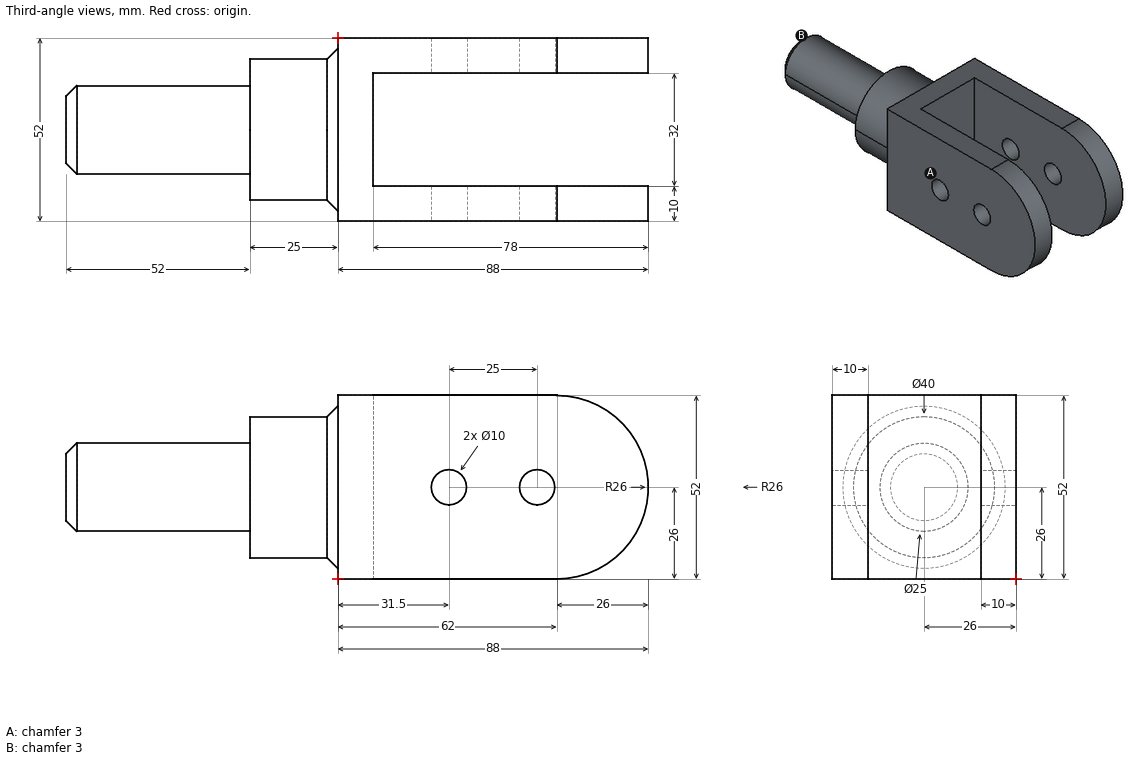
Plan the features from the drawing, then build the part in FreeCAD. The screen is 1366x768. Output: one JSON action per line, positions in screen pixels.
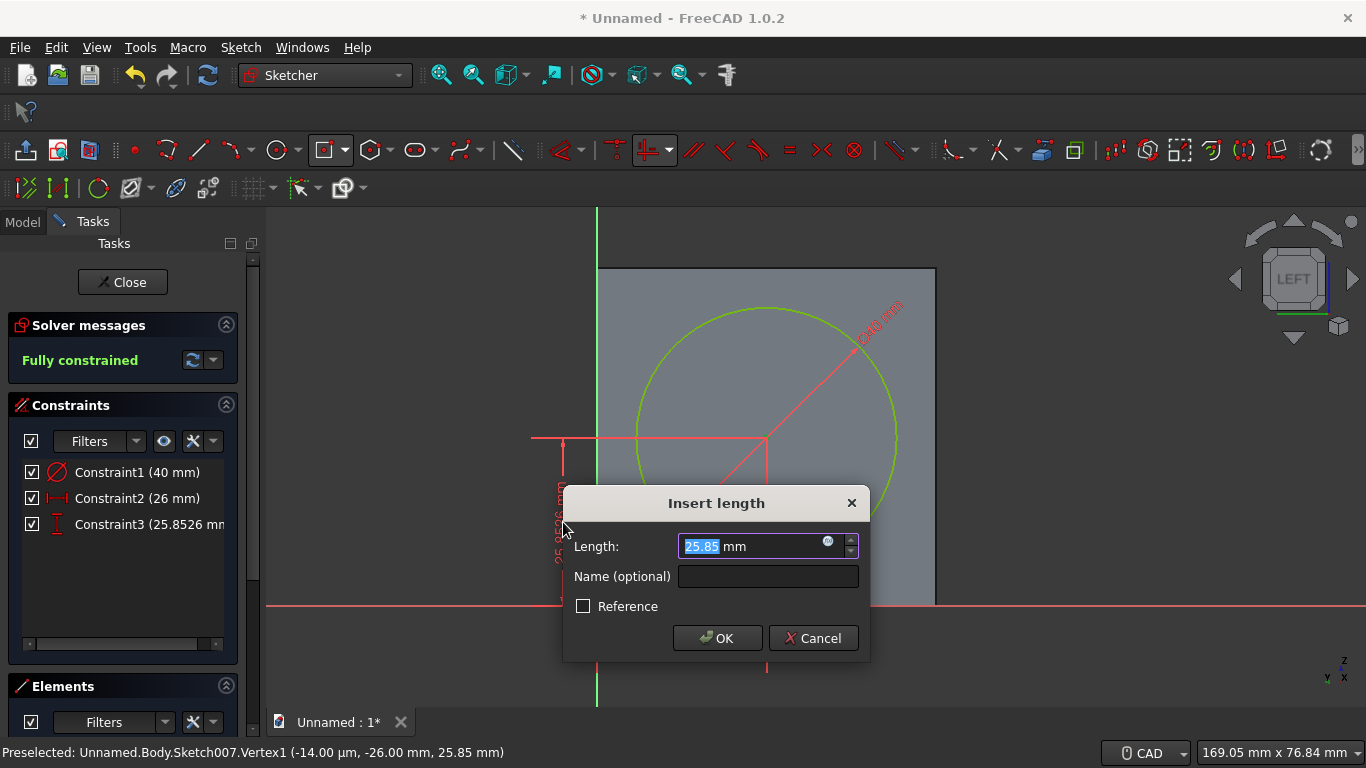
{"action": "type", "text": "26"}
{"action": "key", "text": "Return"}
{"action": "key", "text": "Escape"}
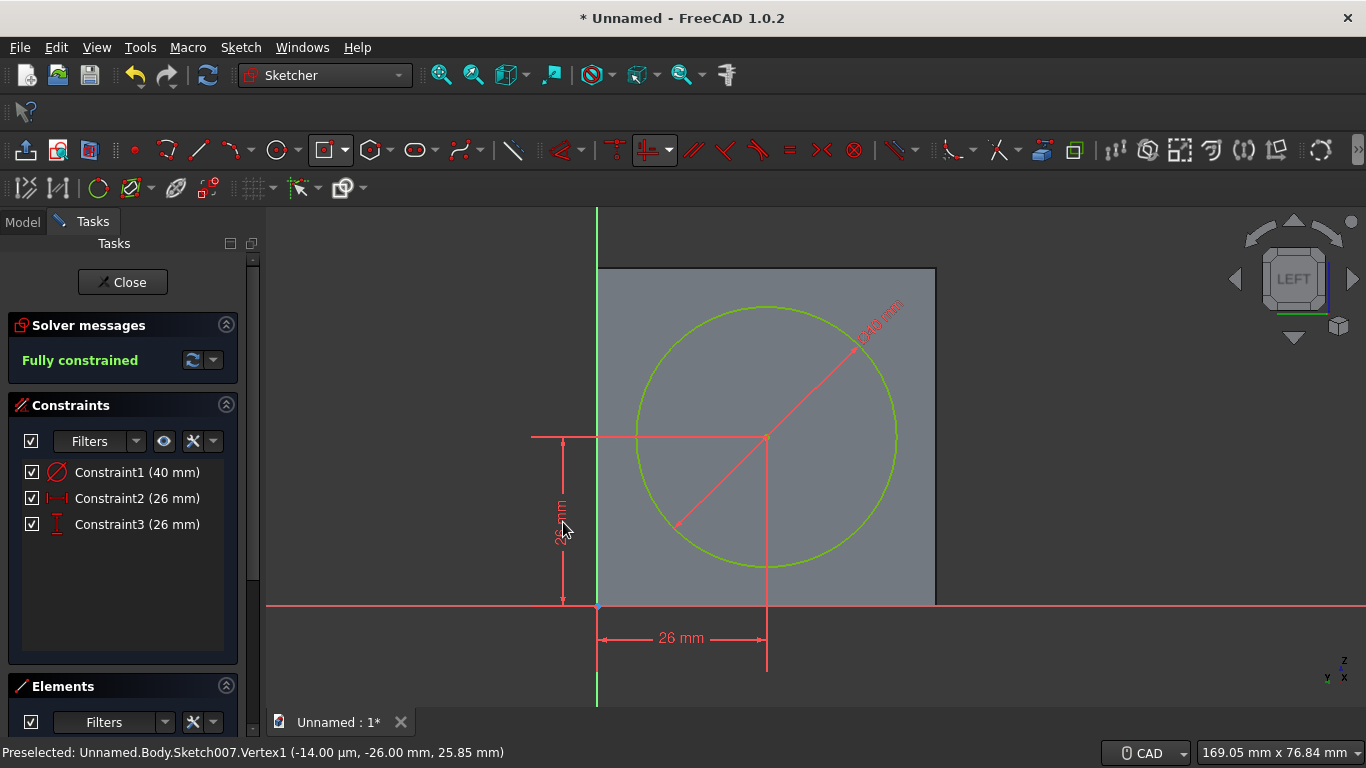
{"action": "left_click", "coordinate": [123, 282]}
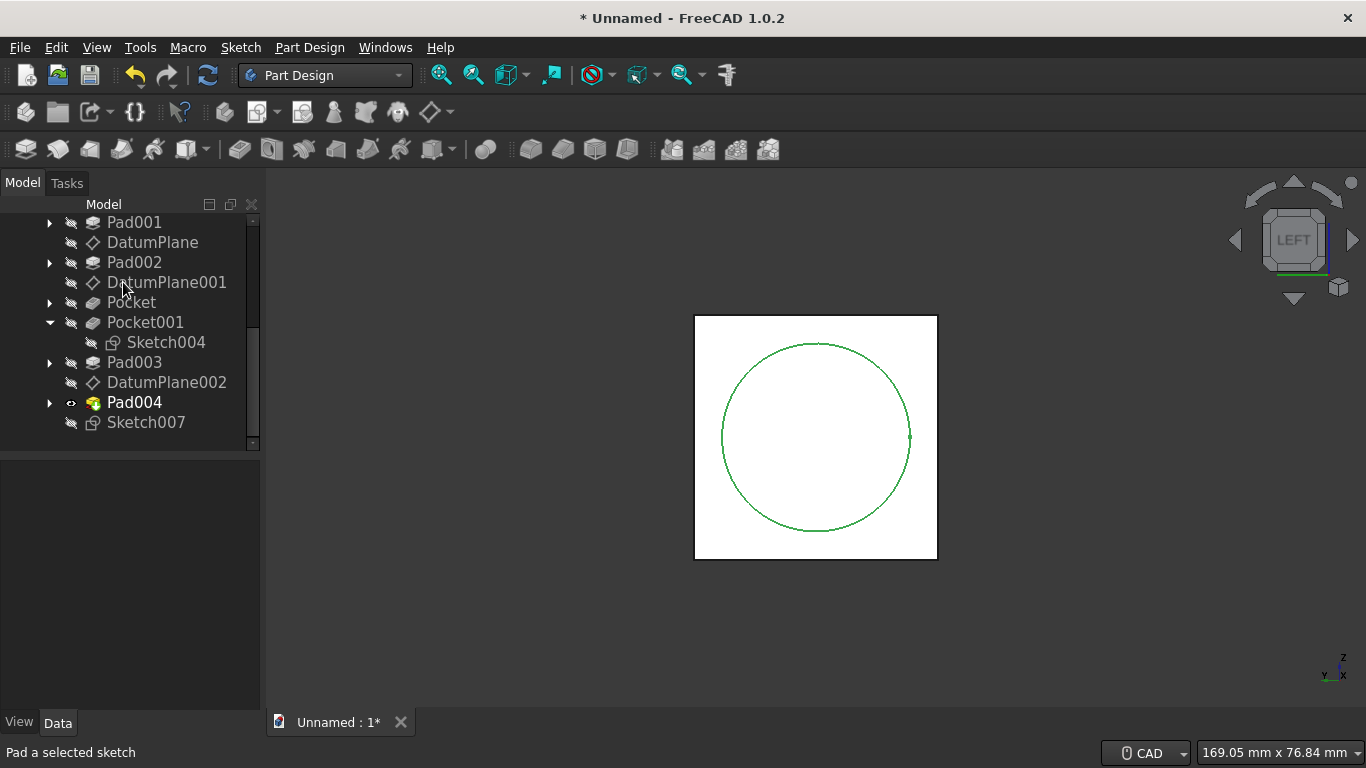
{"action": "left_click", "coordinate": [26, 150]}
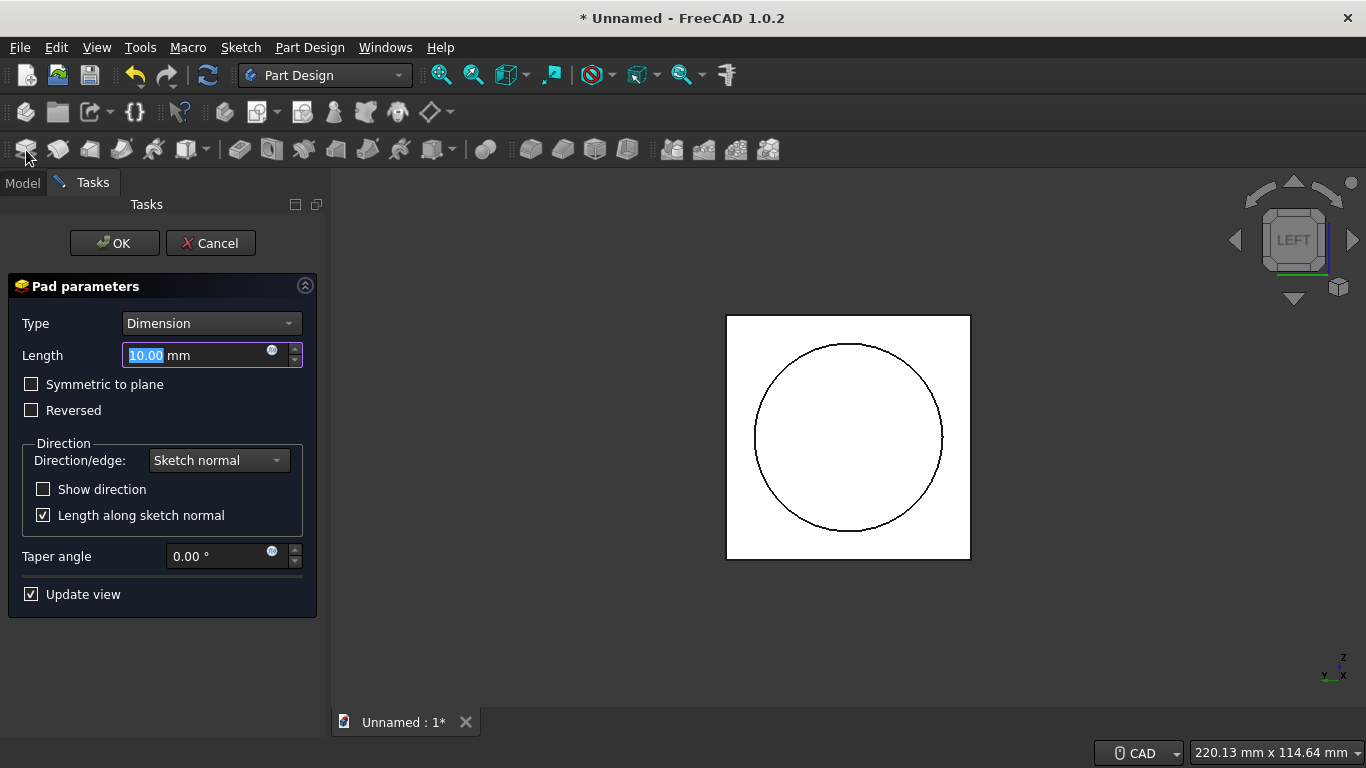
{"action": "type", "text": "25"}
{"action": "key", "text": "Tab"}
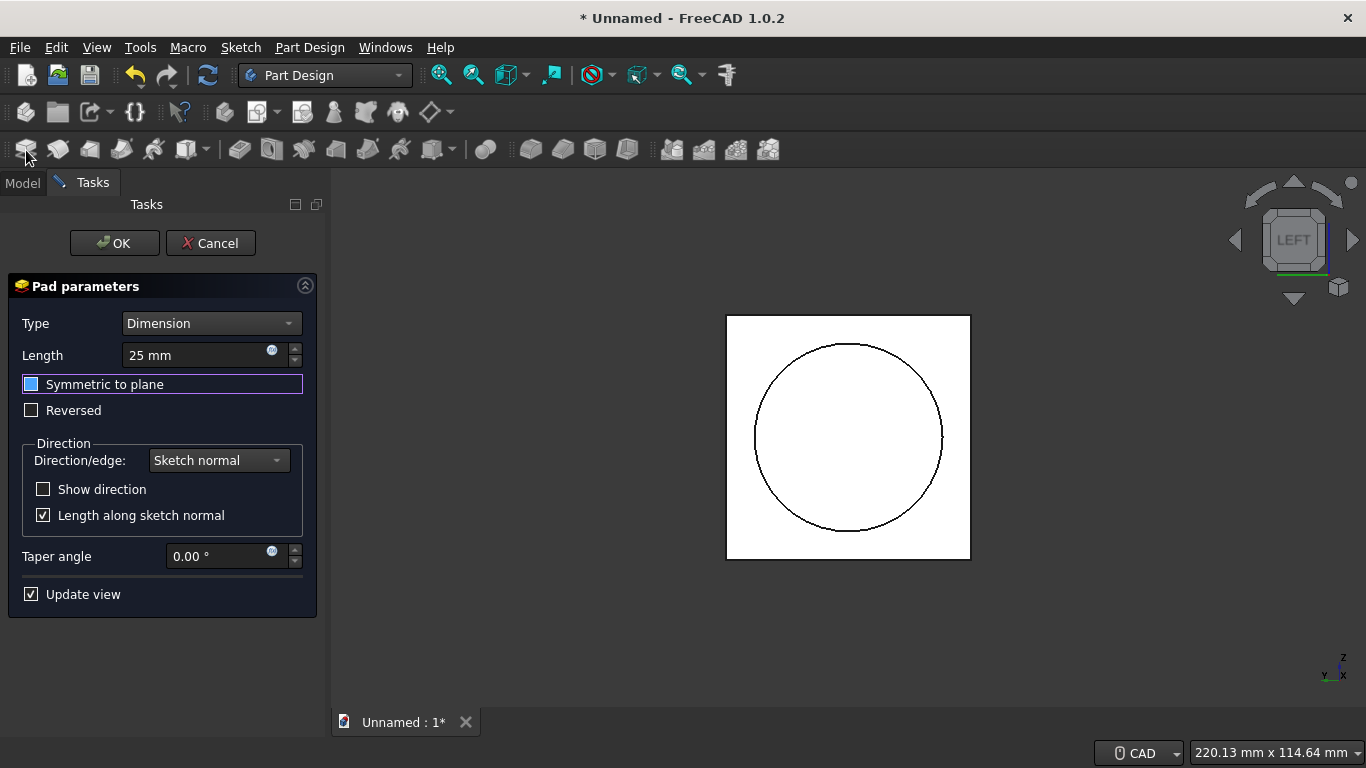
{"action": "left_click", "coordinate": [115, 243]}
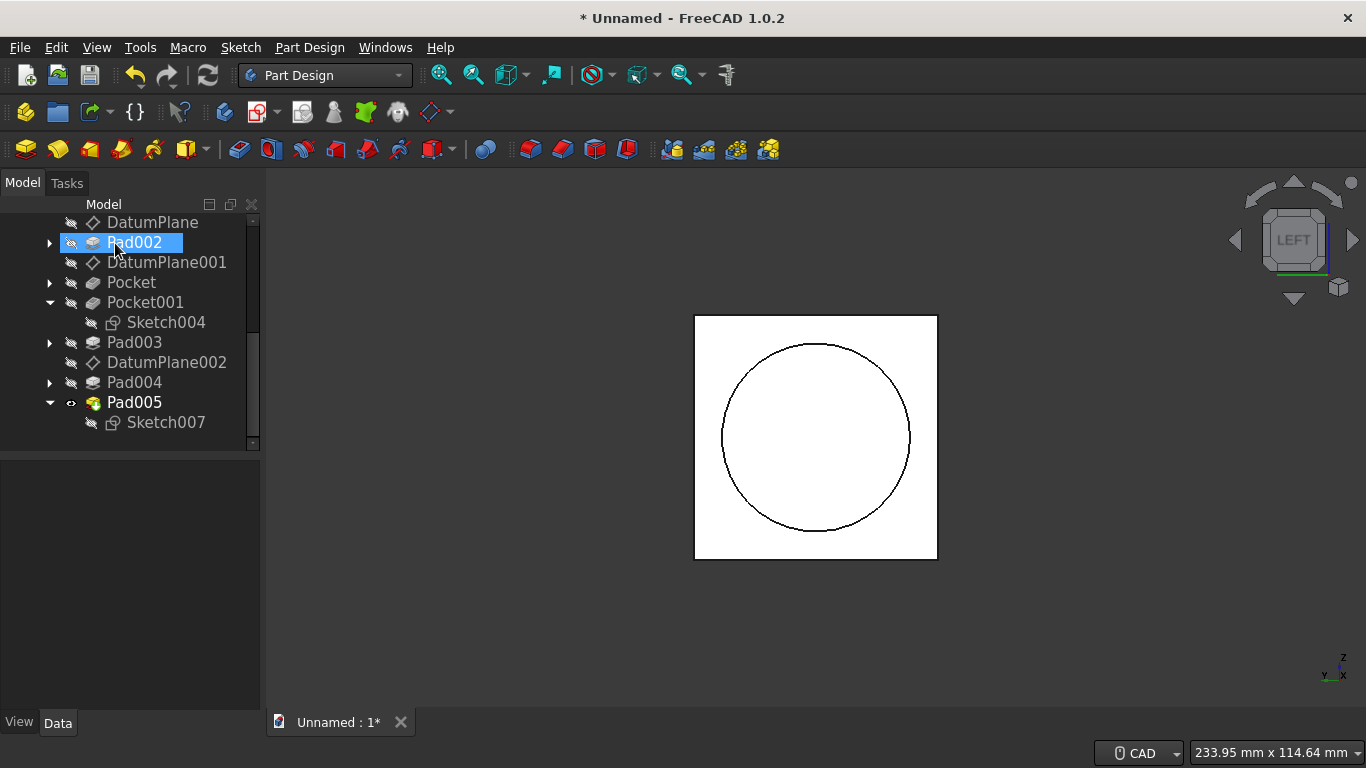
{"action": "key", "text": "0"}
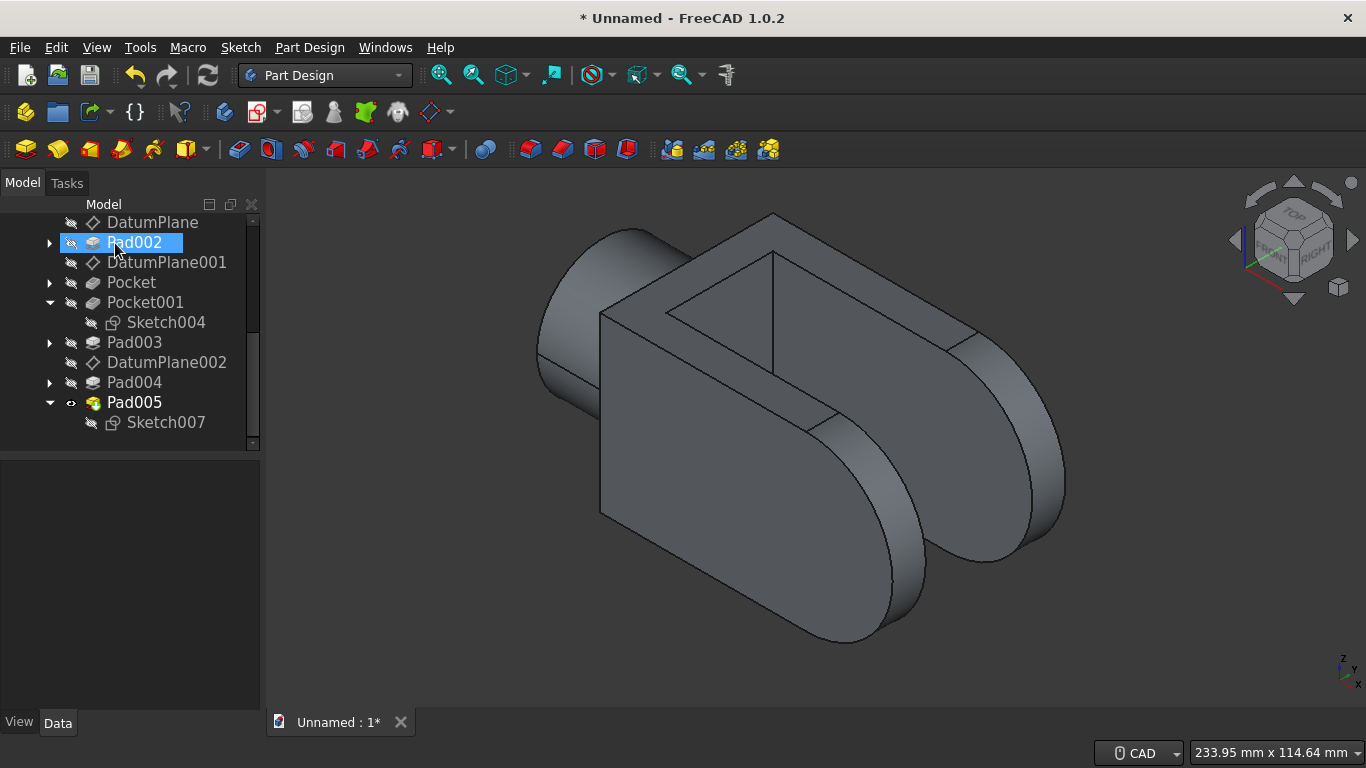
{"action": "left_click", "coordinate": [442, 76]}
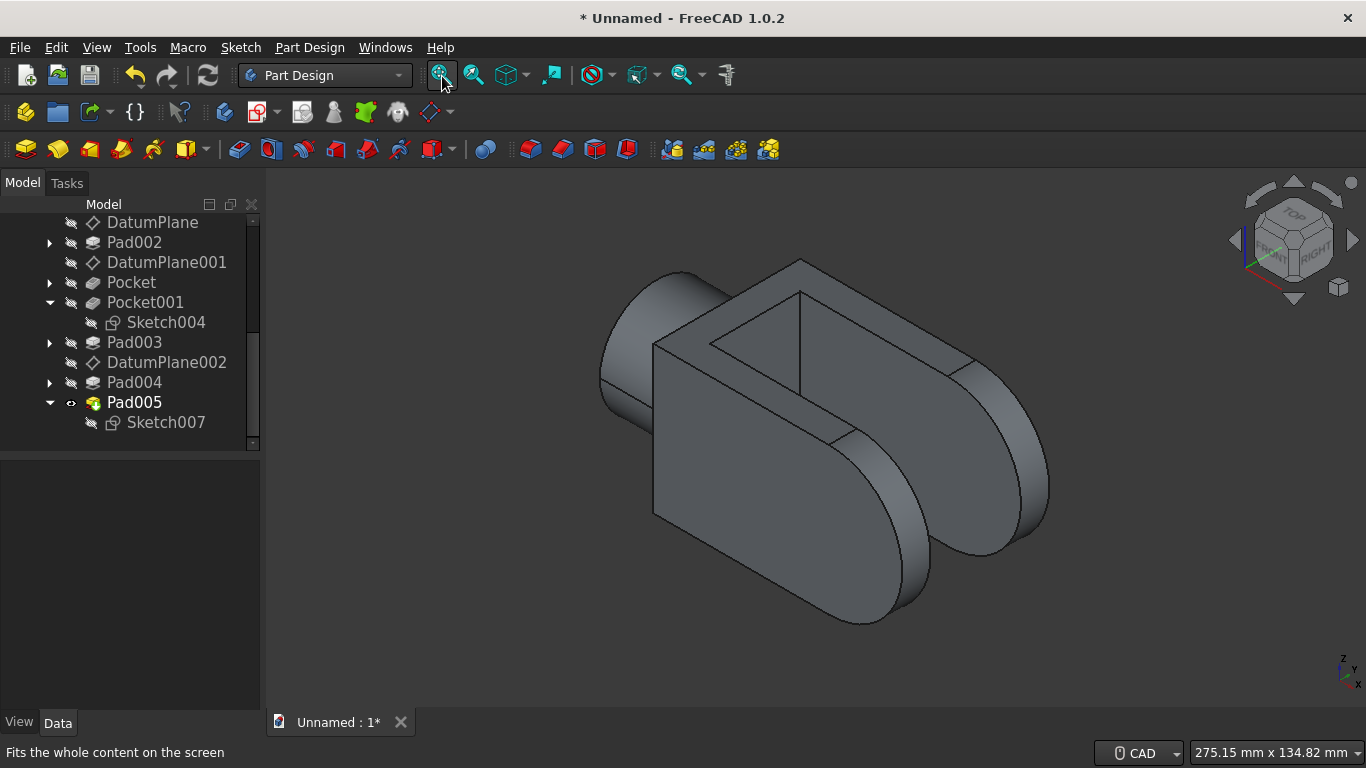
{"action": "key", "text": "2"}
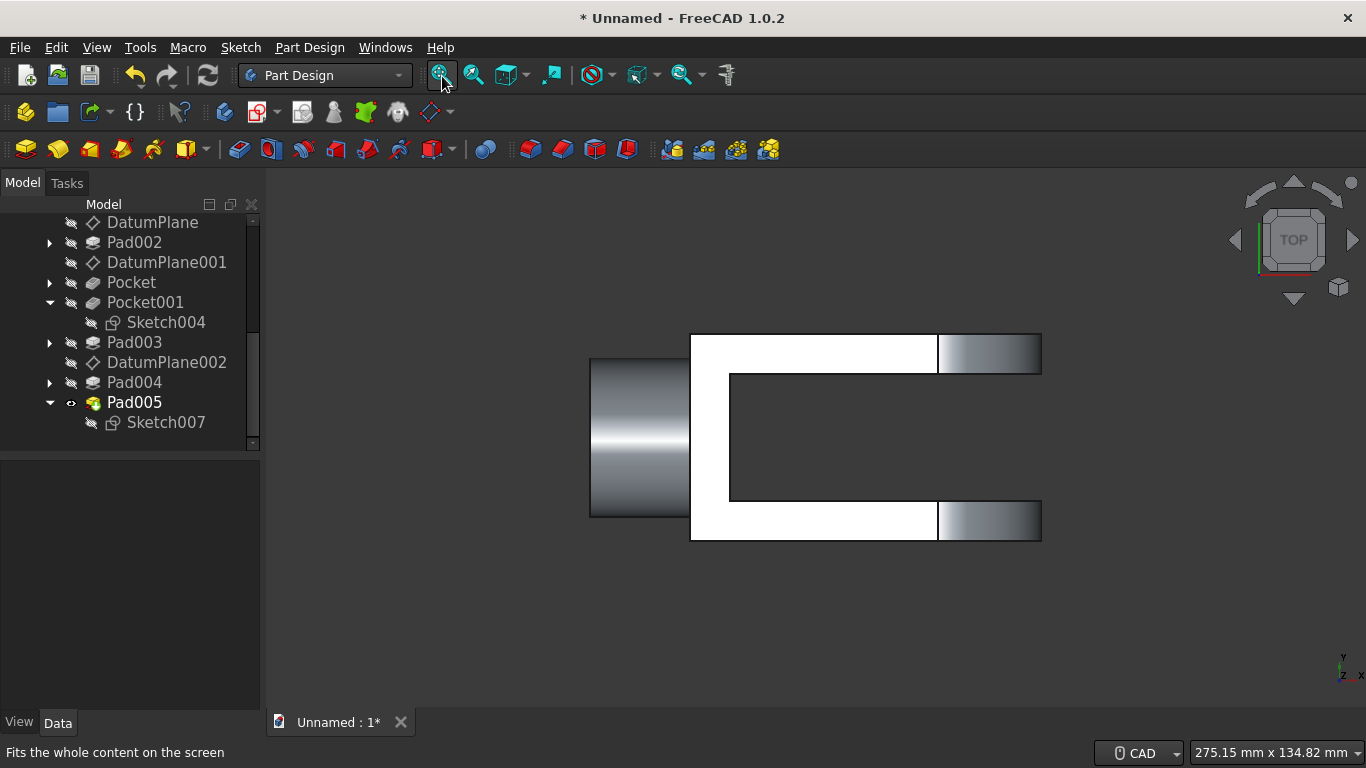
{"action": "left_click", "coordinate": [442, 76]}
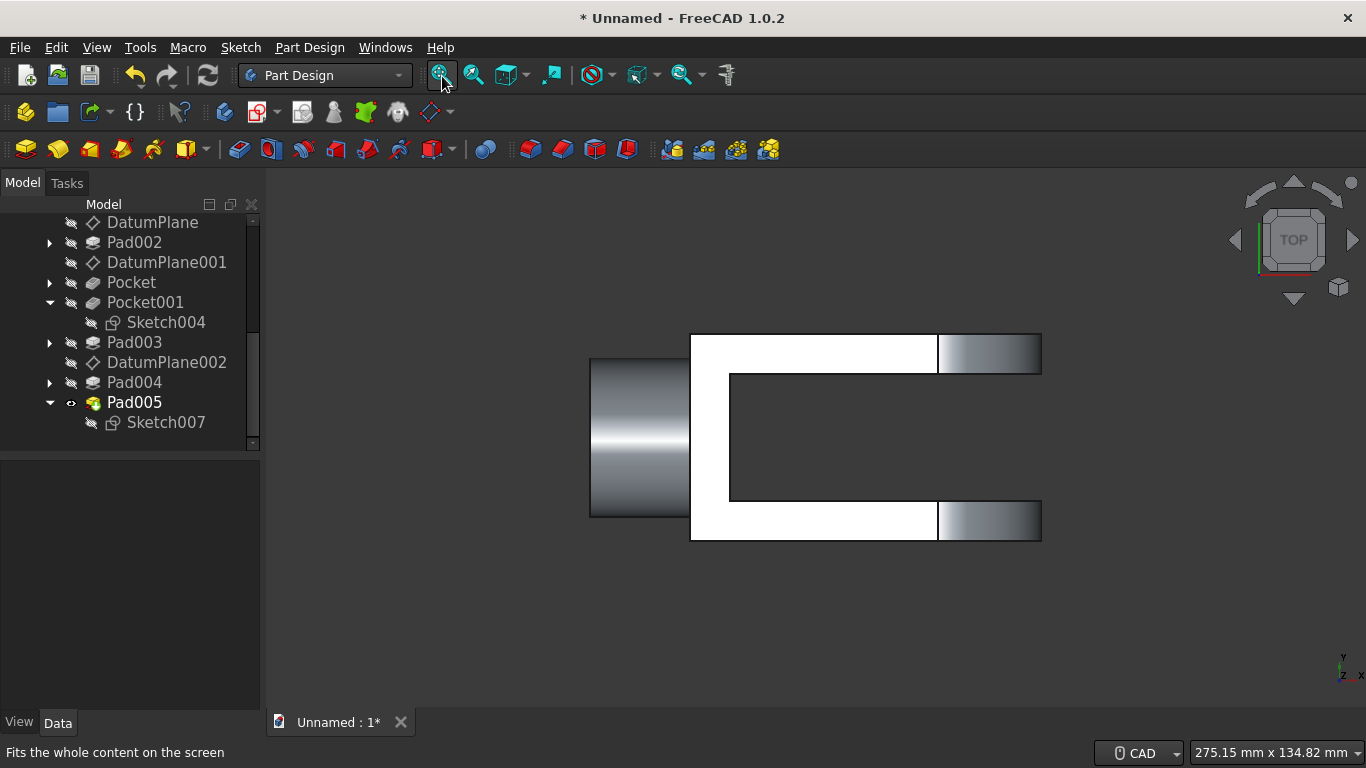
{"action": "key", "text": "1"}